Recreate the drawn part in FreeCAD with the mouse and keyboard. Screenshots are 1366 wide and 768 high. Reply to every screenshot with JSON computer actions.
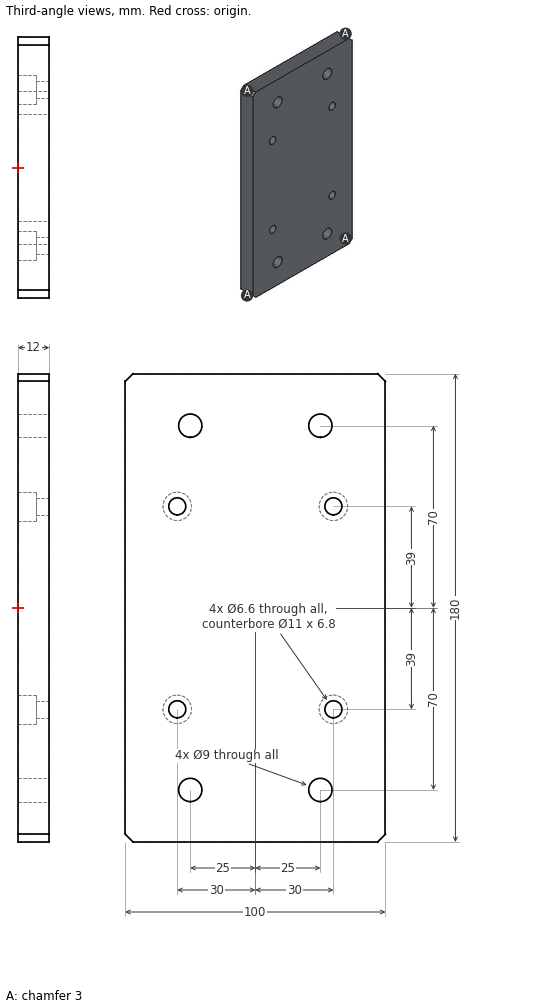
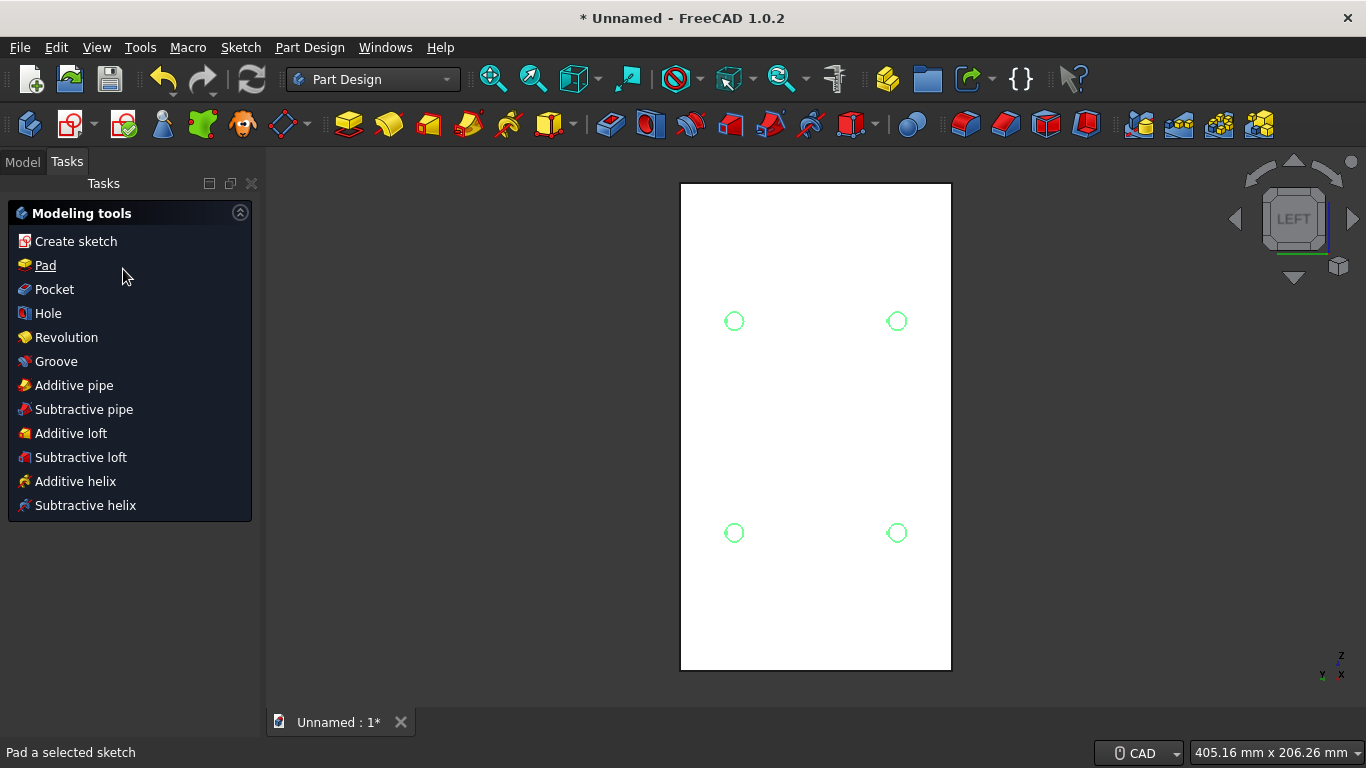
{"action": "left_click", "coordinate": [652, 124]}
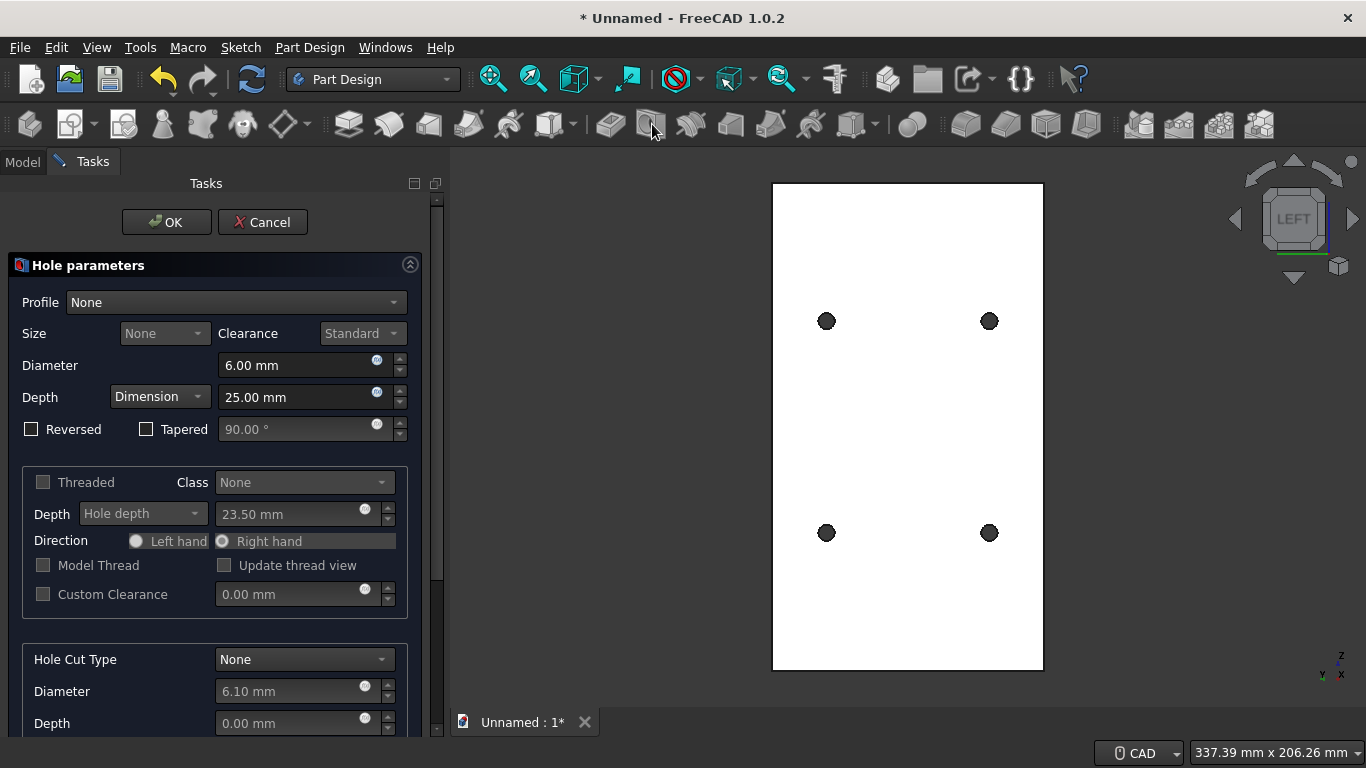
{"action": "triple_click", "coordinate": [305, 365]}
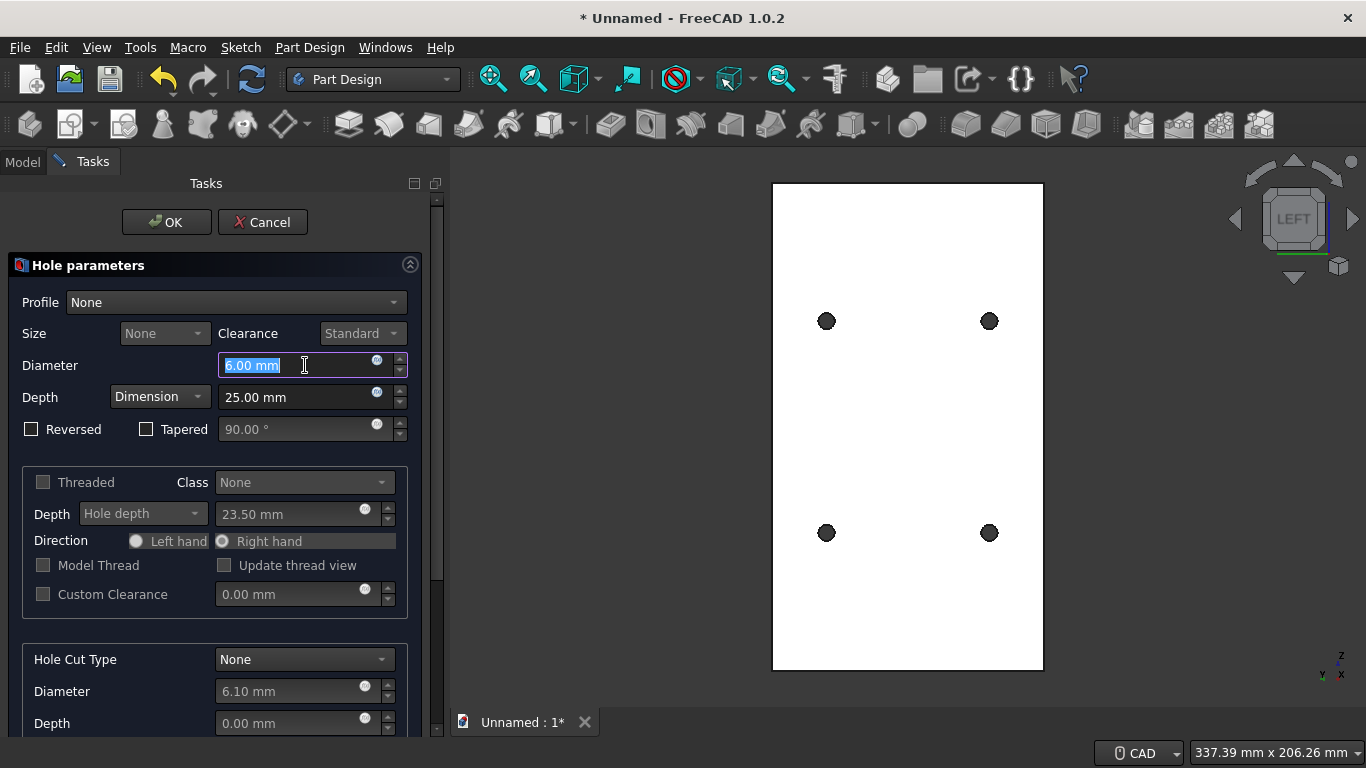
{"action": "type", "text": "6.6"}
{"action": "key", "text": "Tab"}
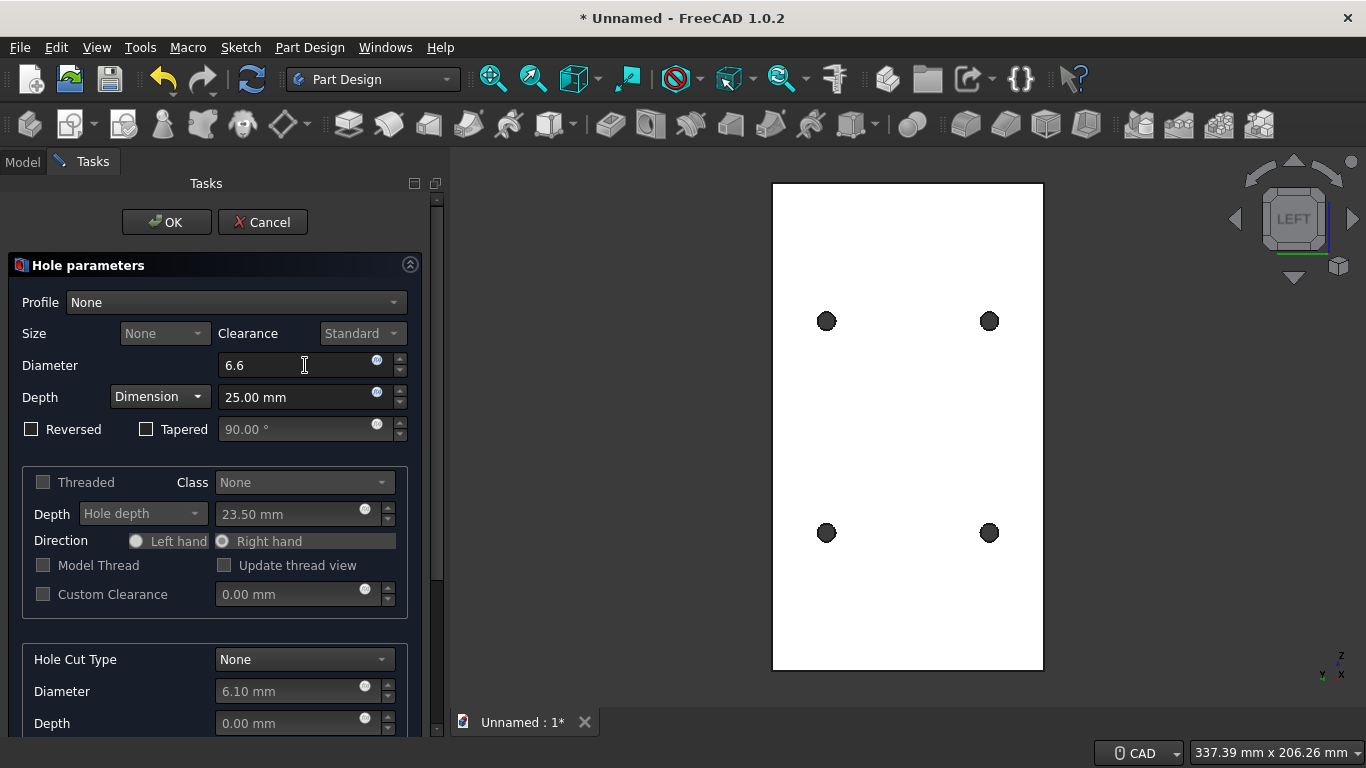
{"action": "left_click", "coordinate": [161, 396]}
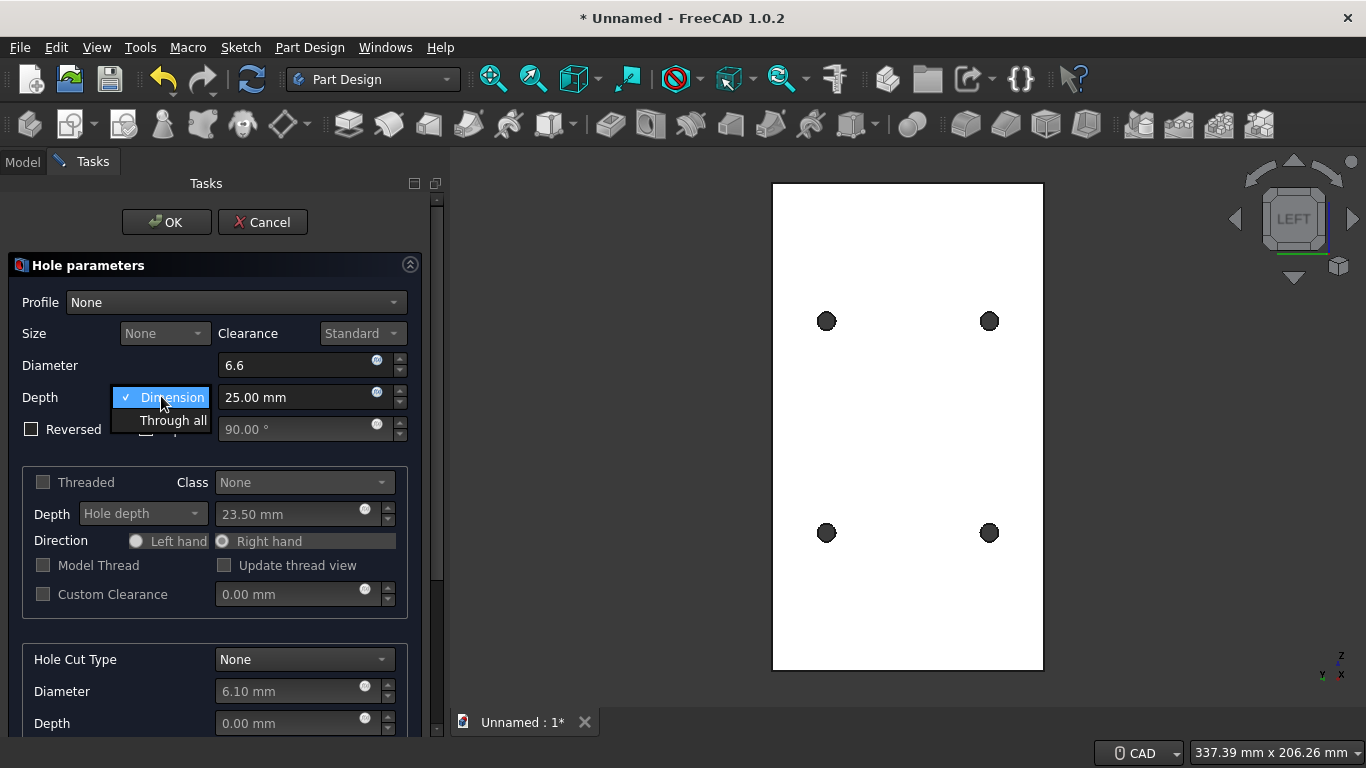
{"action": "left_click", "coordinate": [160, 420]}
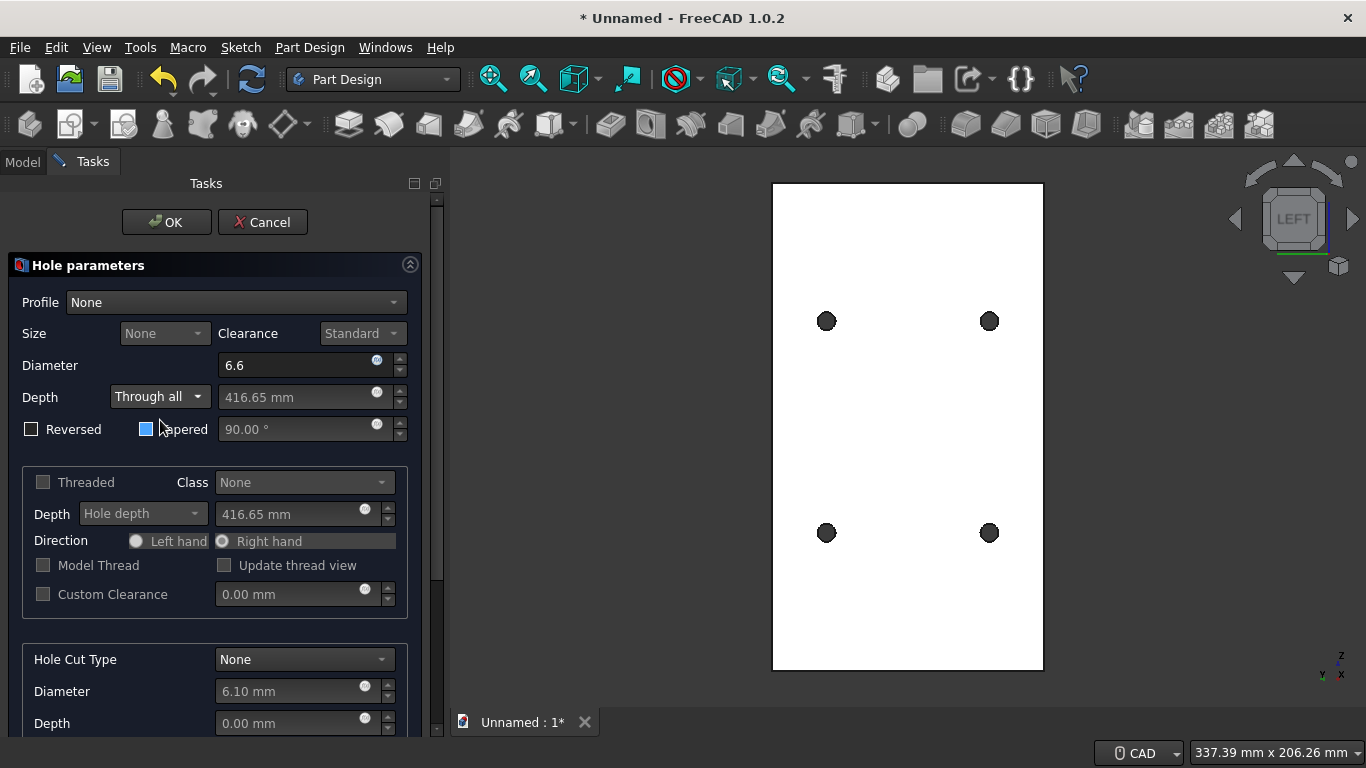
{"action": "left_click", "coordinate": [306, 660]}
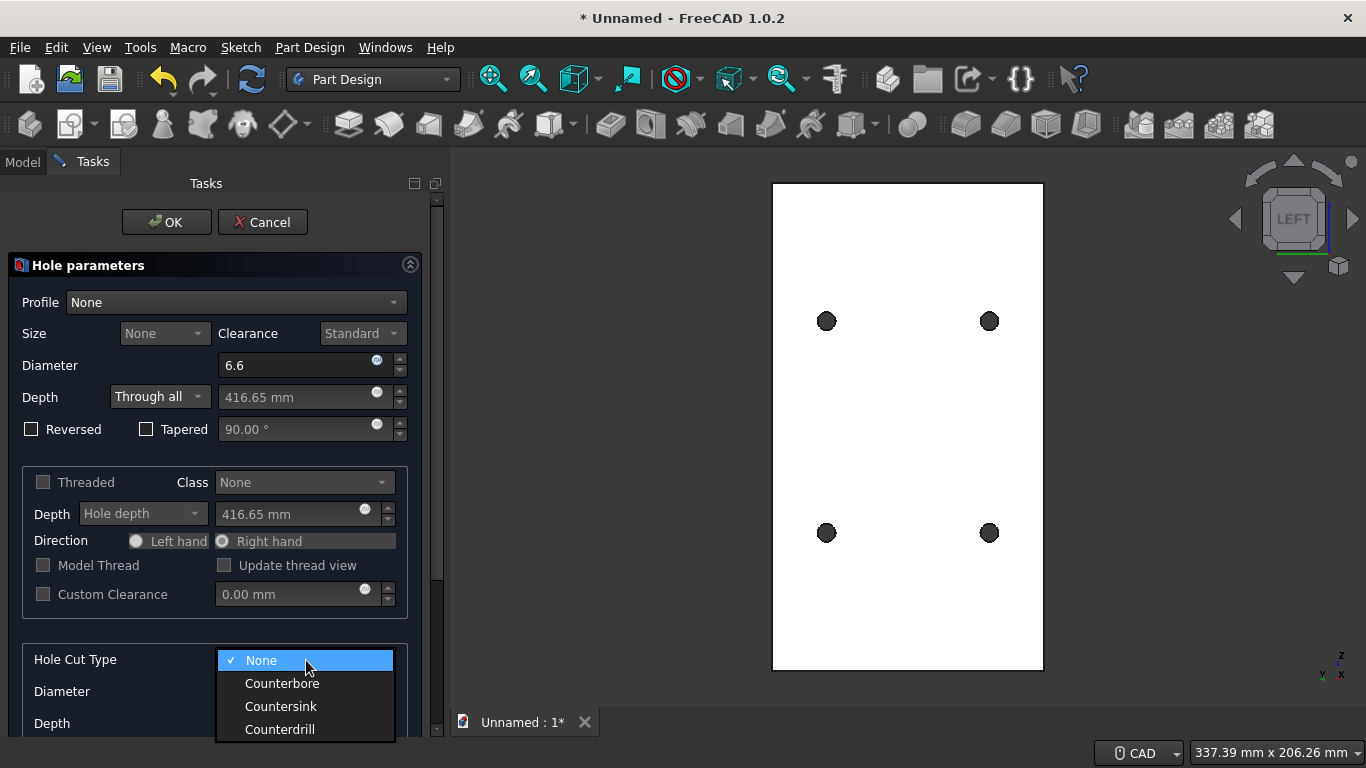
{"action": "left_click", "coordinate": [304, 684]}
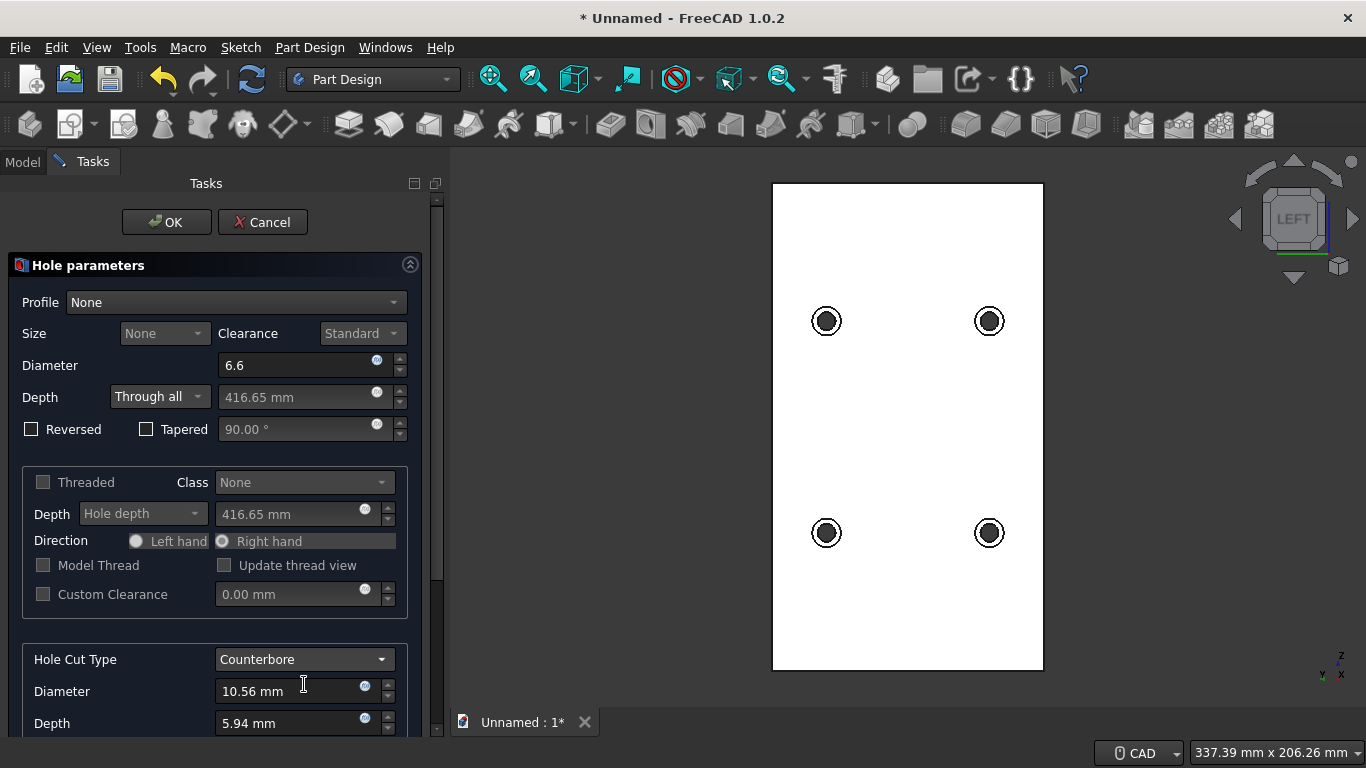
{"action": "triple_click", "coordinate": [298, 691]}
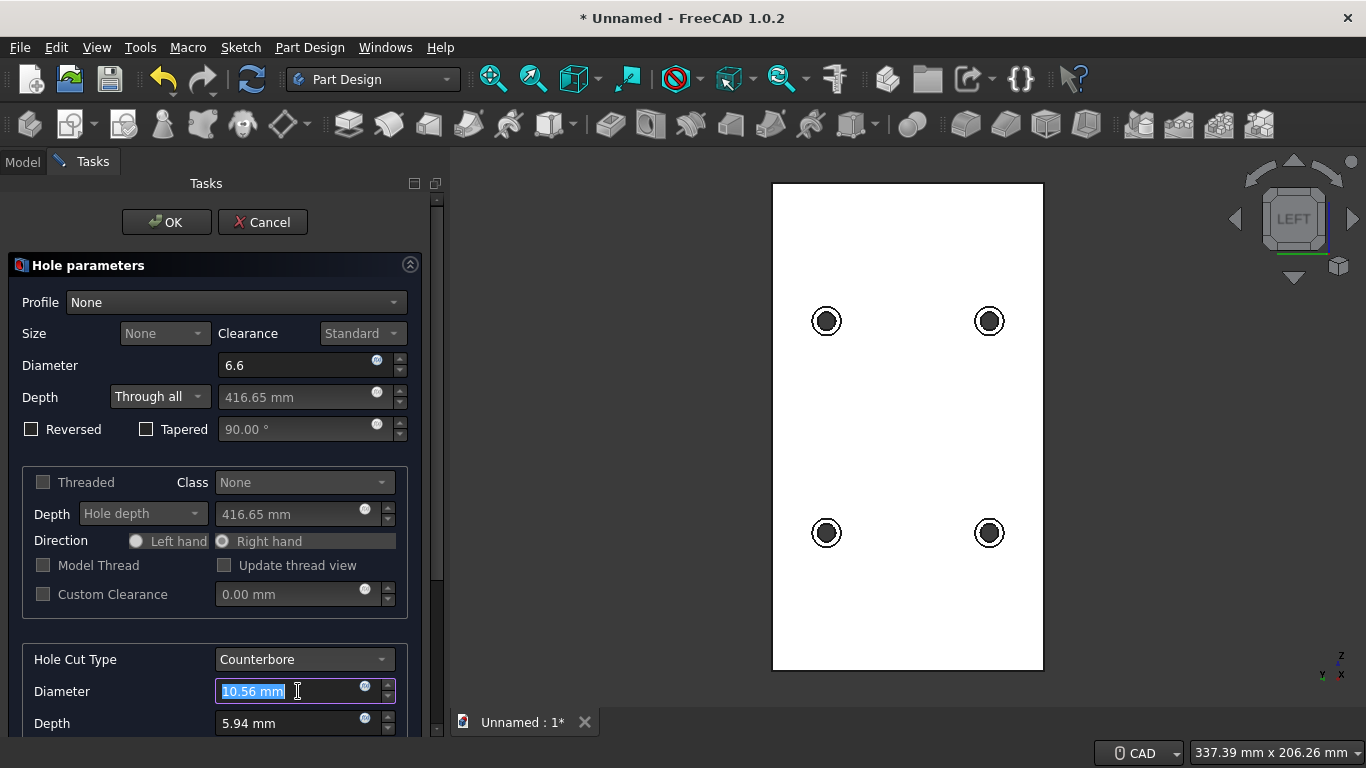
{"action": "type", "text": "11"}
{"action": "key", "text": "Tab"}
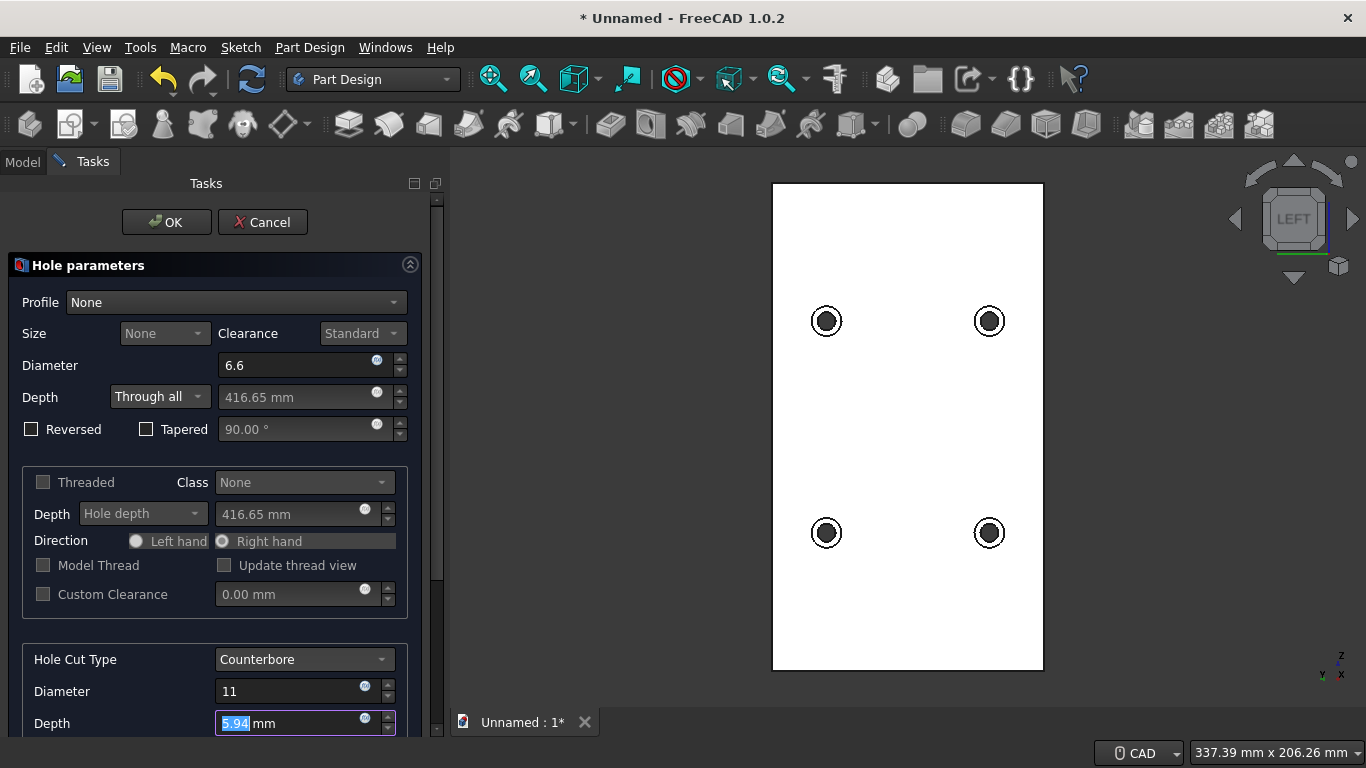
{"action": "type", "text": "6.8"}
{"action": "key", "text": "Tab"}